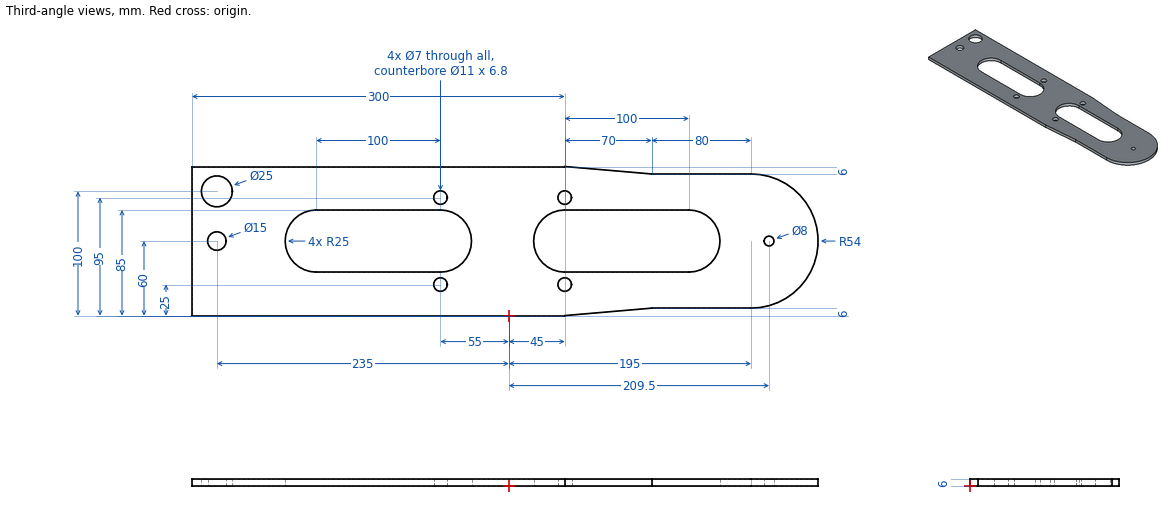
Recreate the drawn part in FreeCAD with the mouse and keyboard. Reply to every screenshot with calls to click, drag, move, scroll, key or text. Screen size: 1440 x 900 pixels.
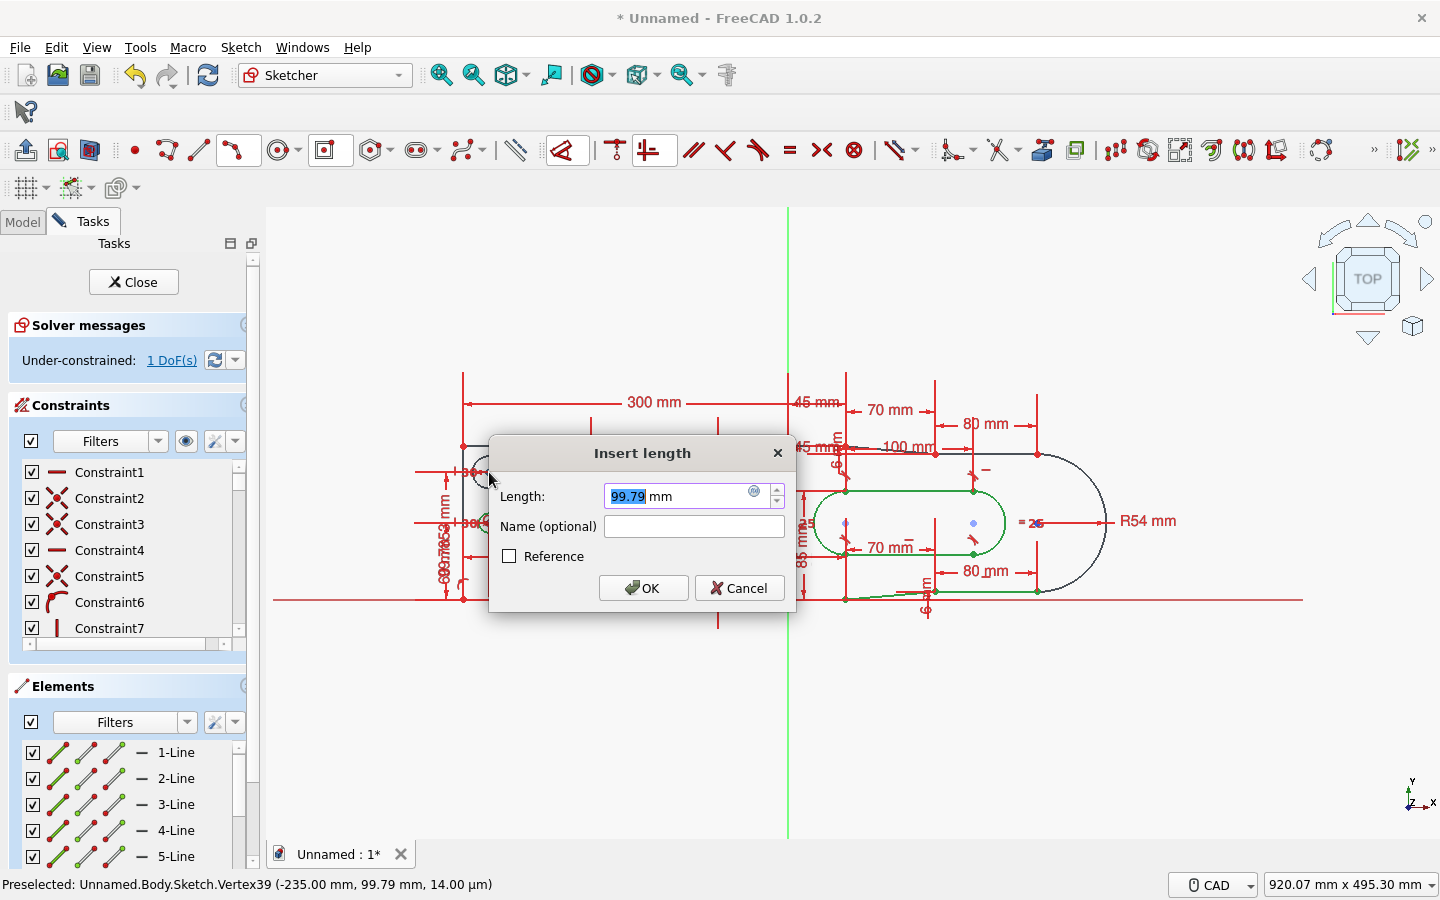
text(100)
key(Return)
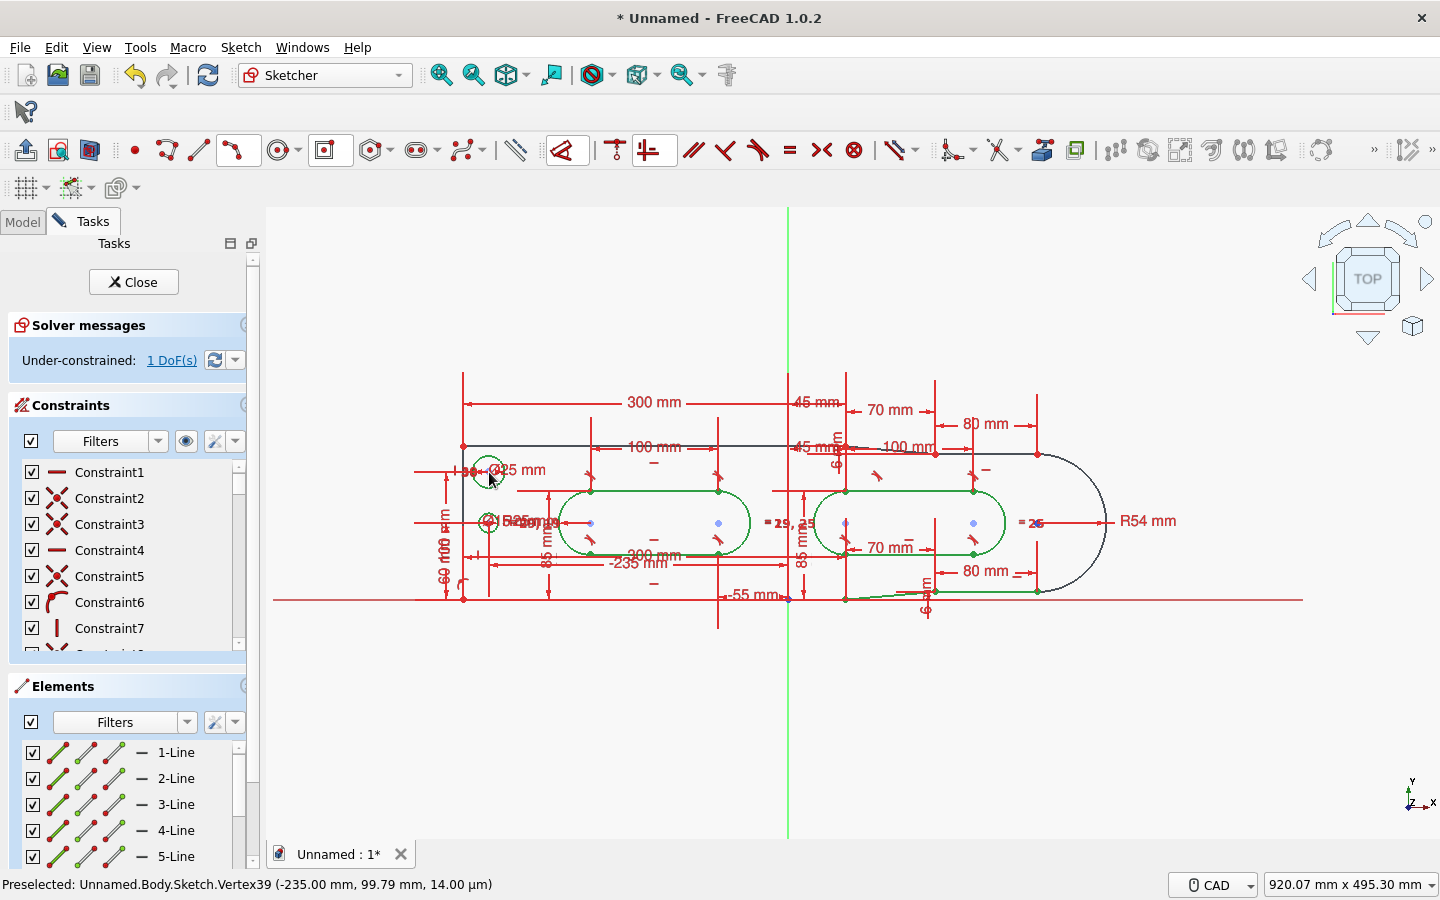
scroll(1037, 523, up, 4)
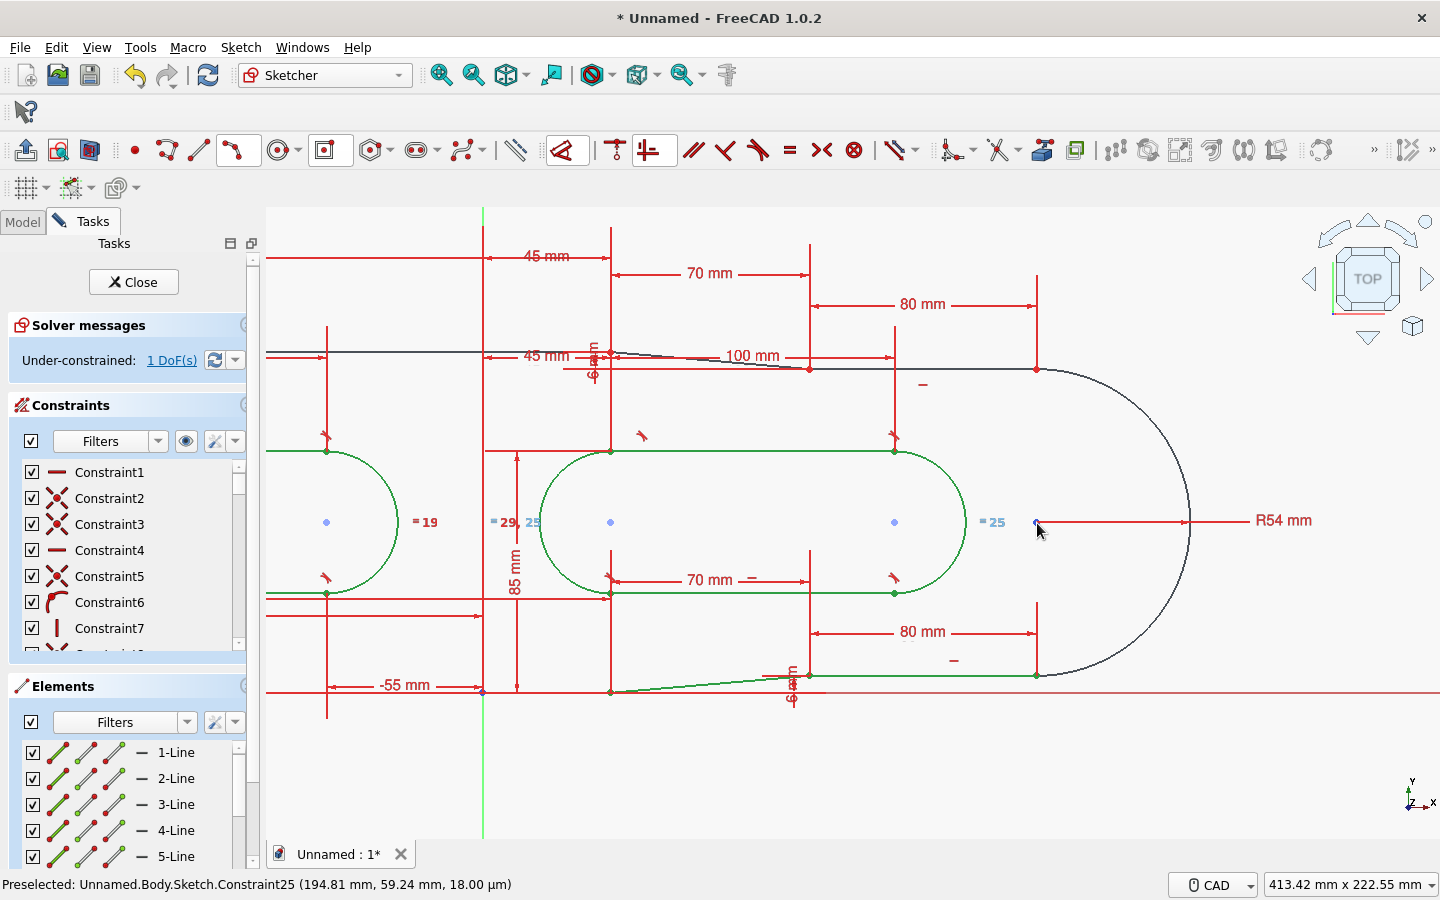
click(1037, 522)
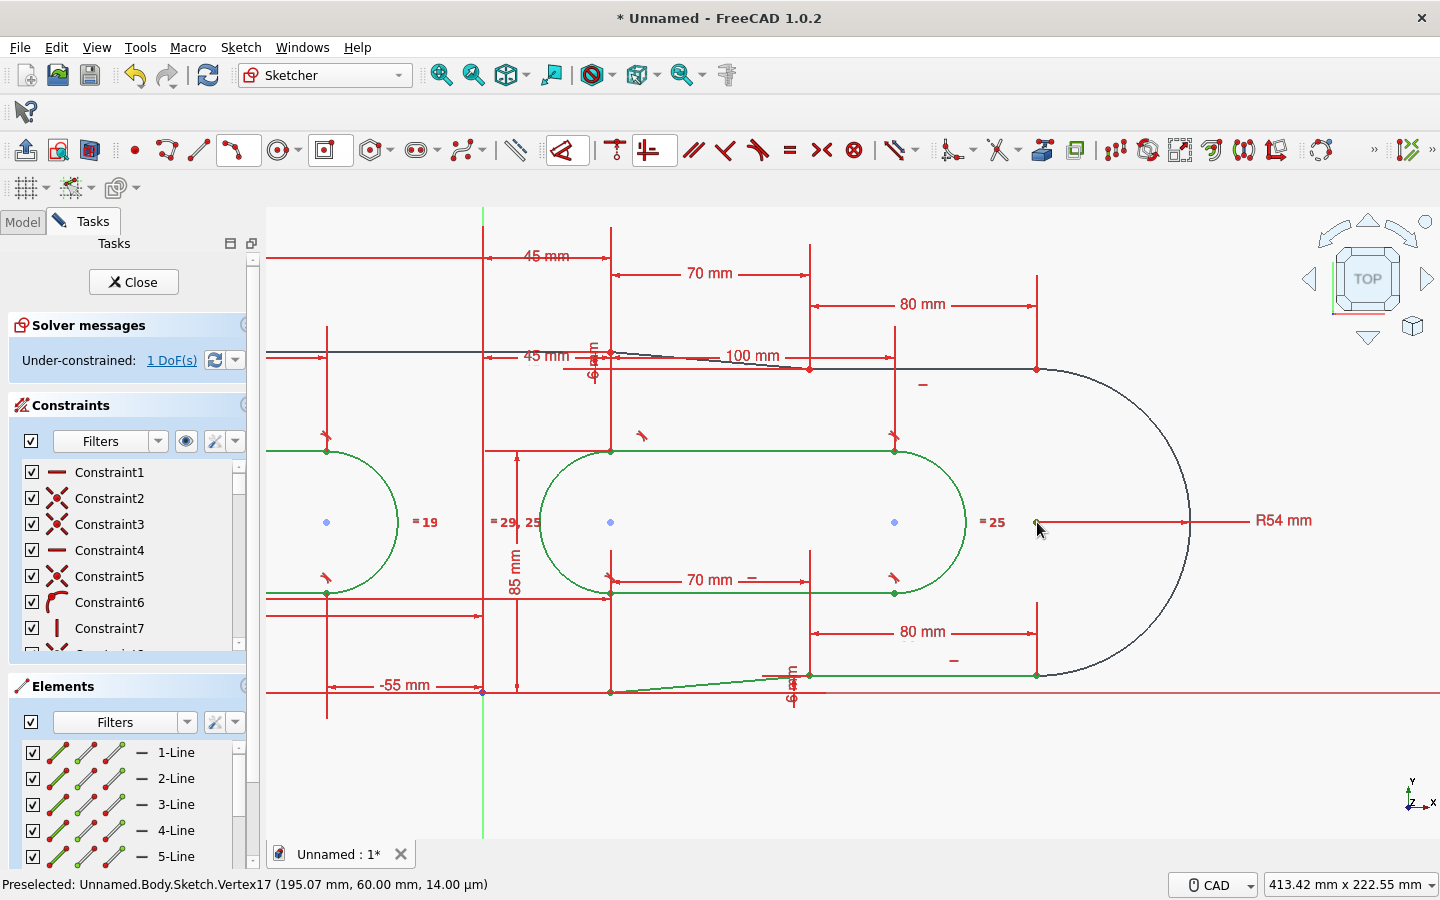
key(l)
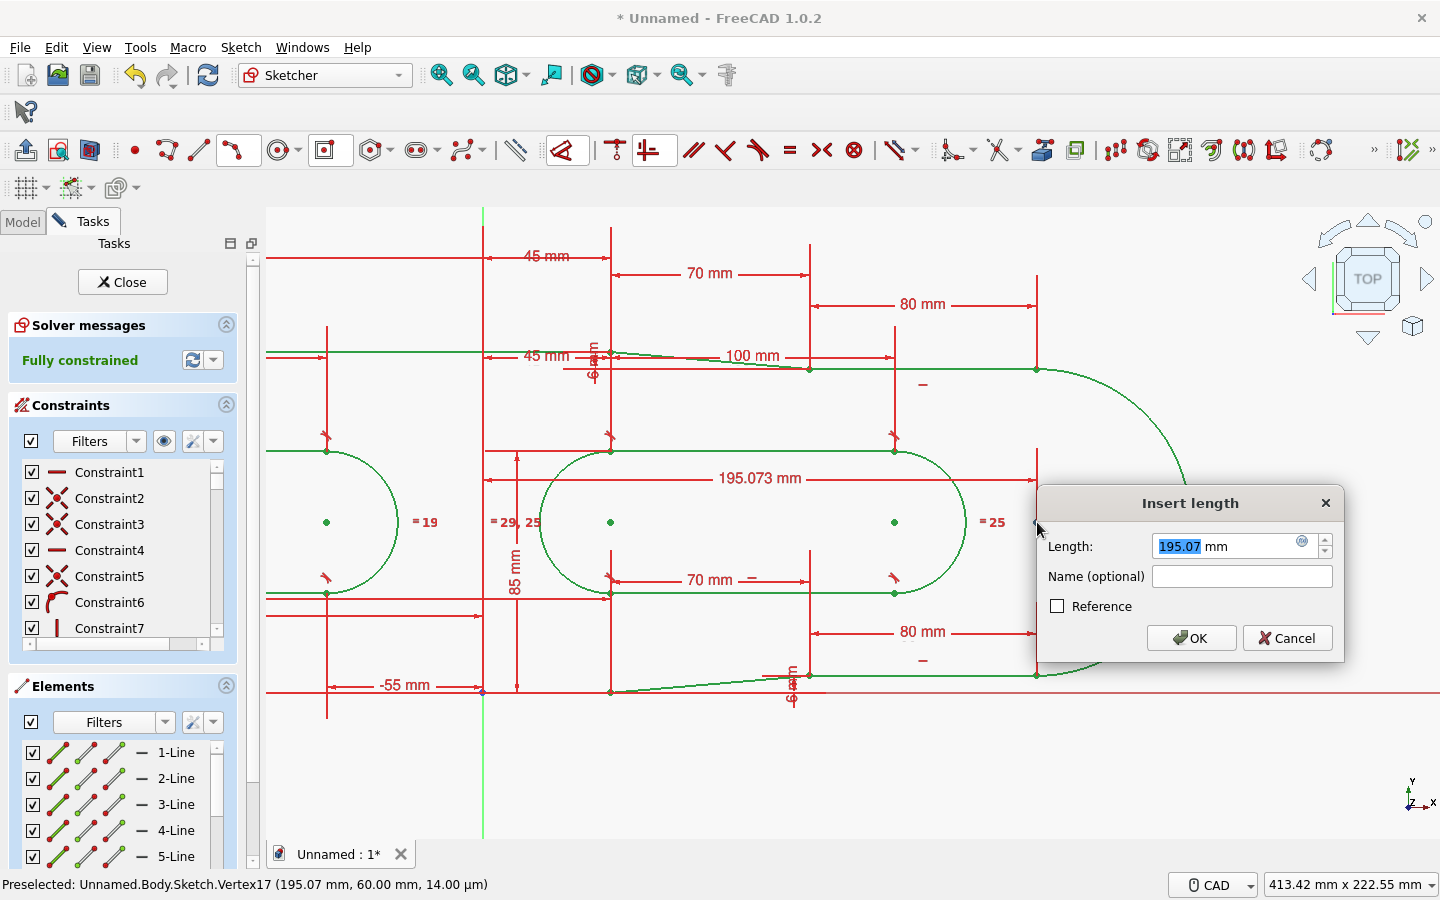
text(195)
key(Return)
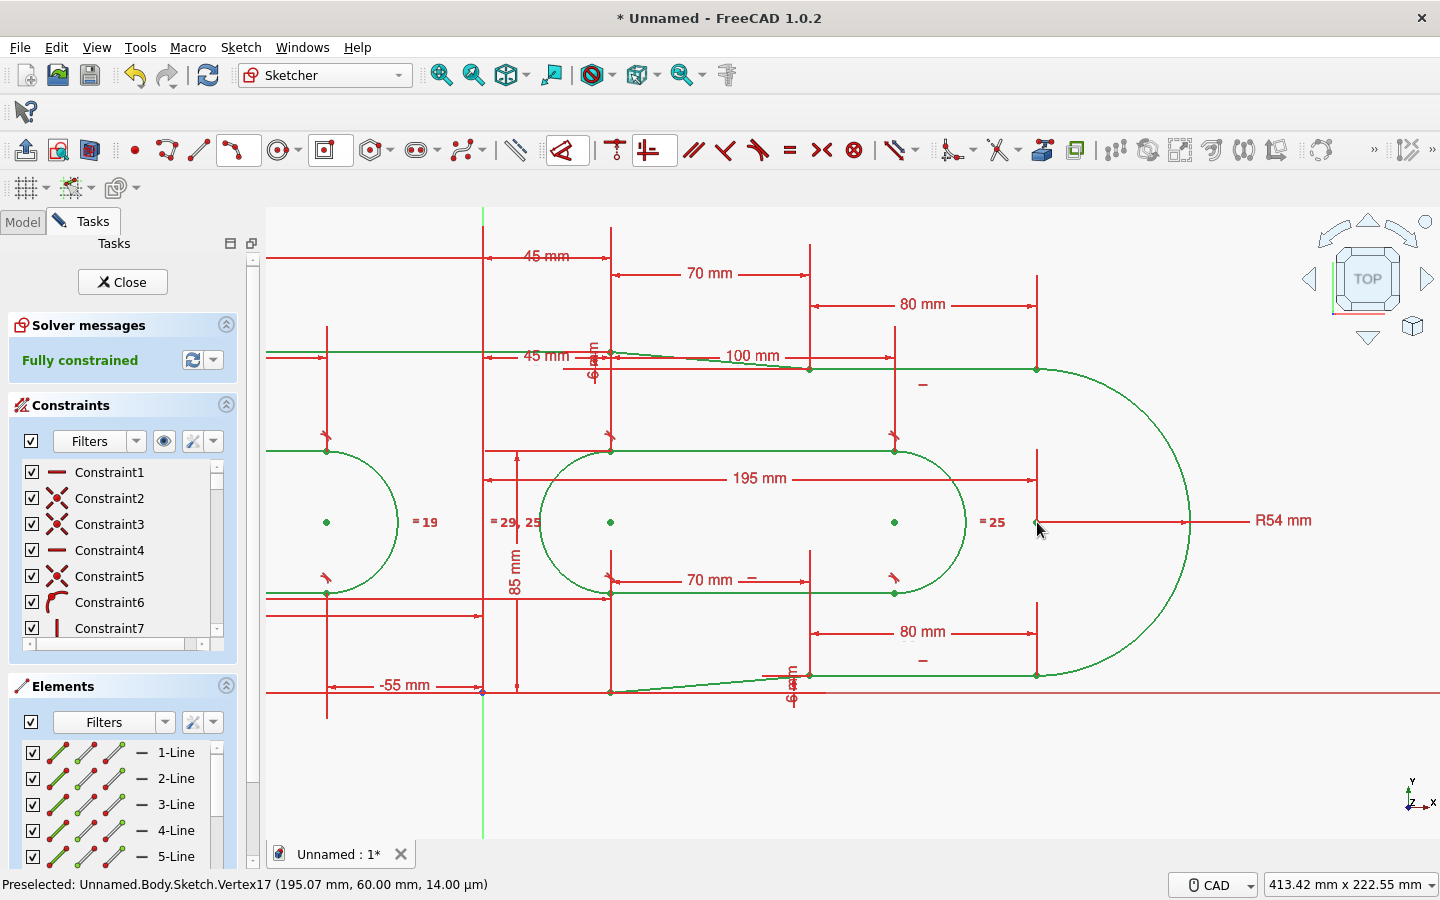
click(123, 282)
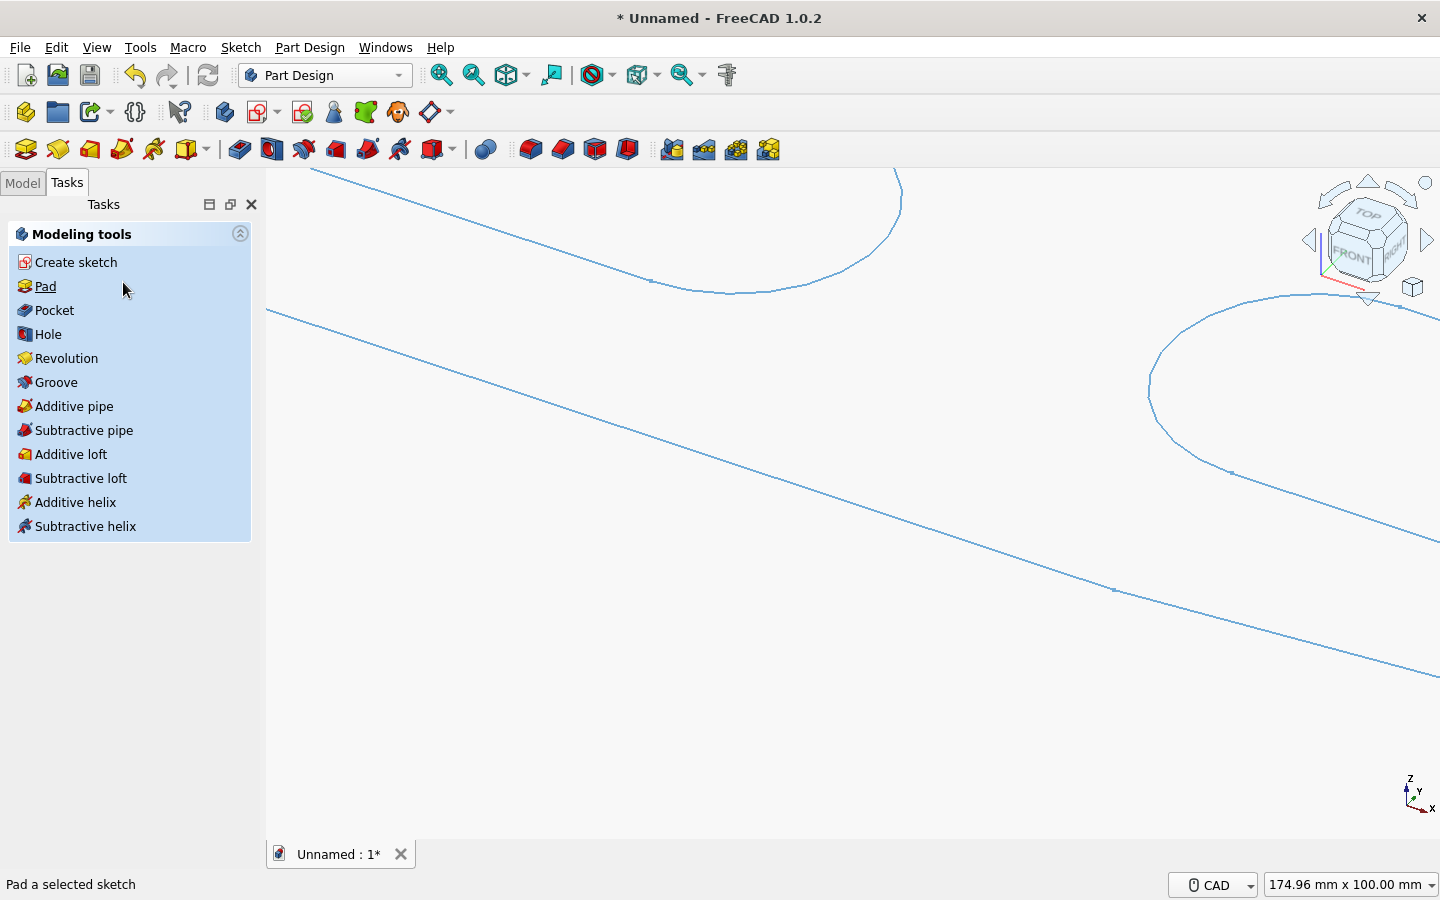
click(26, 150)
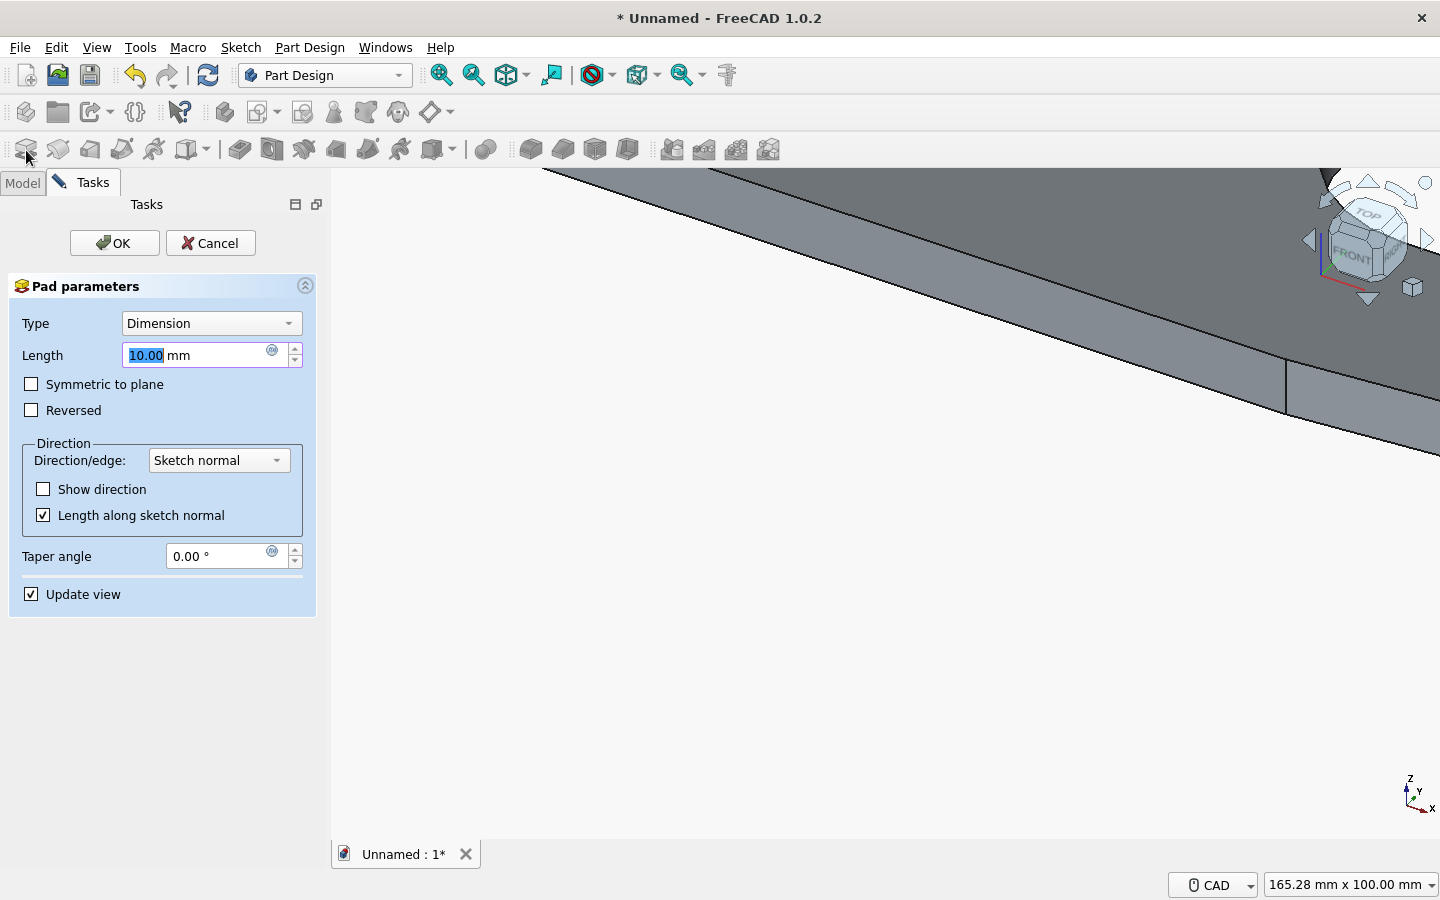
text(6)
key(Tab)